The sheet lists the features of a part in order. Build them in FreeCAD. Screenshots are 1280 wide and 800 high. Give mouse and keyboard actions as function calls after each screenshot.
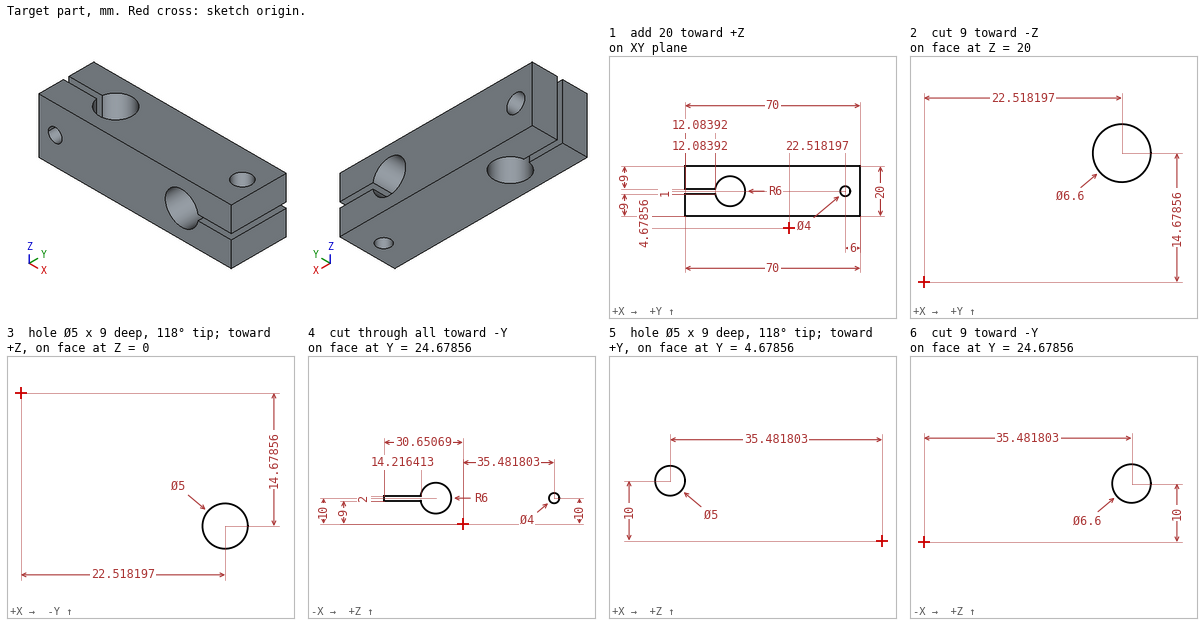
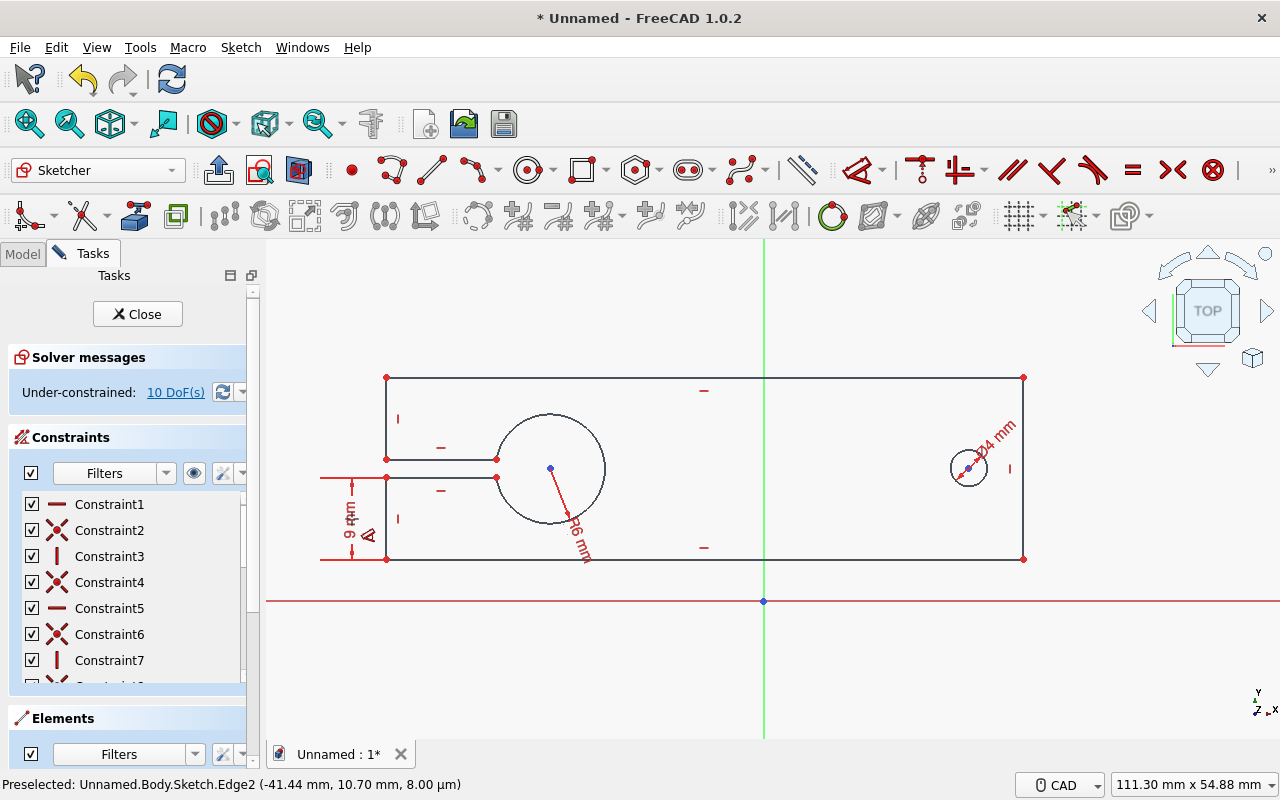
click(386, 403)
click(352, 419)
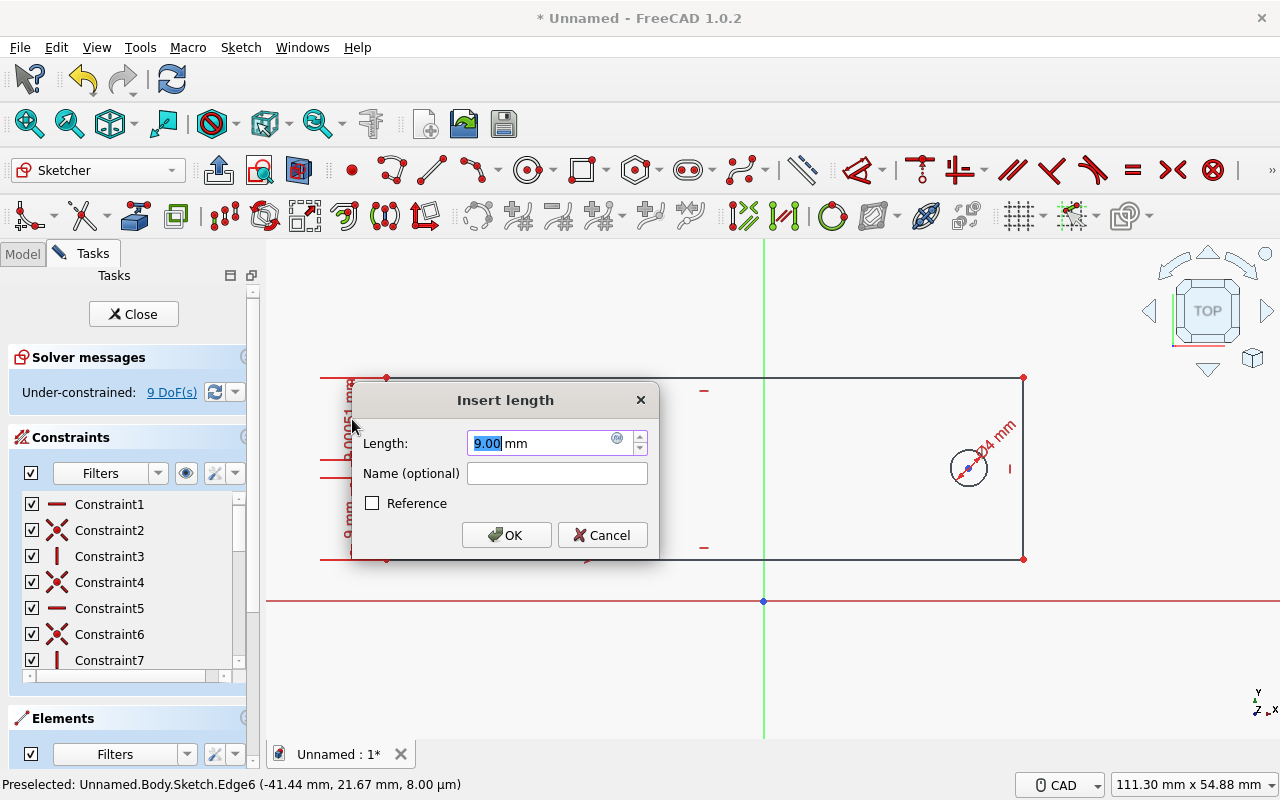
text(9)
key(Return)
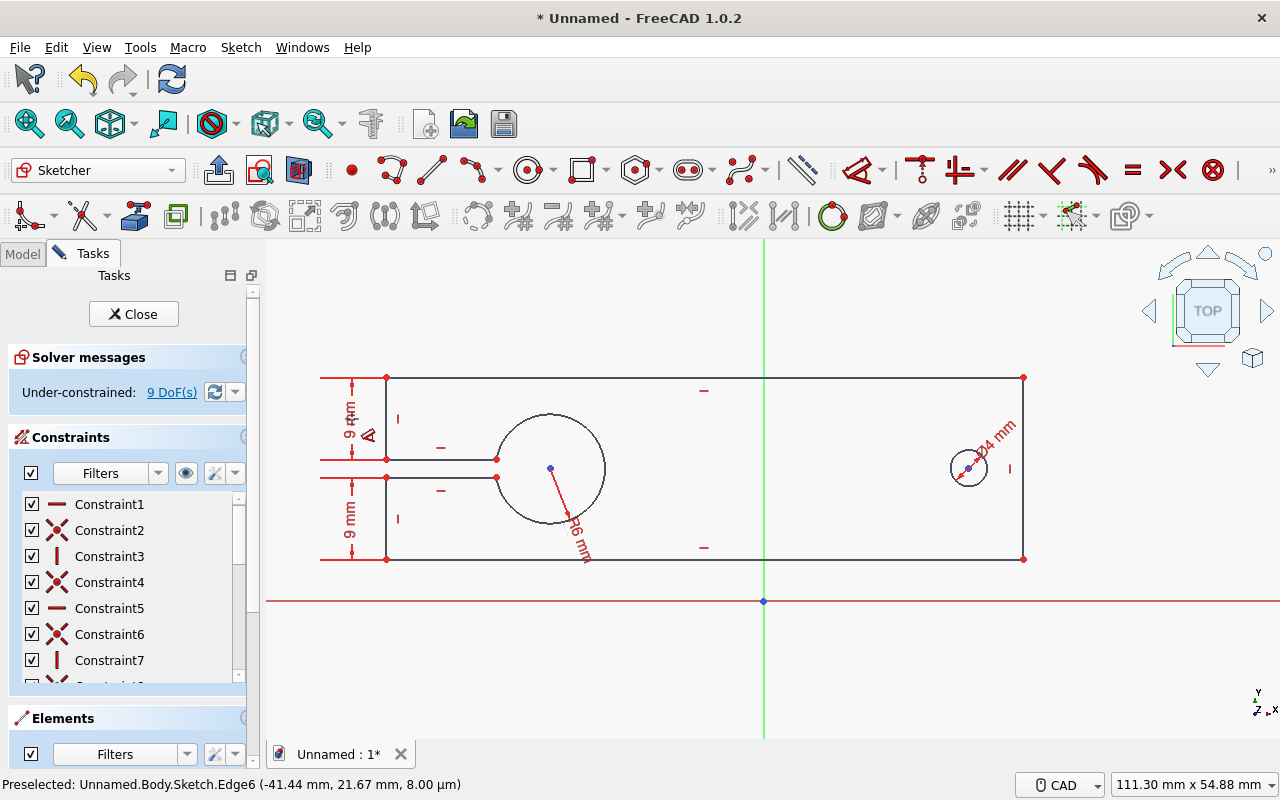
click(577, 560)
click(705, 526)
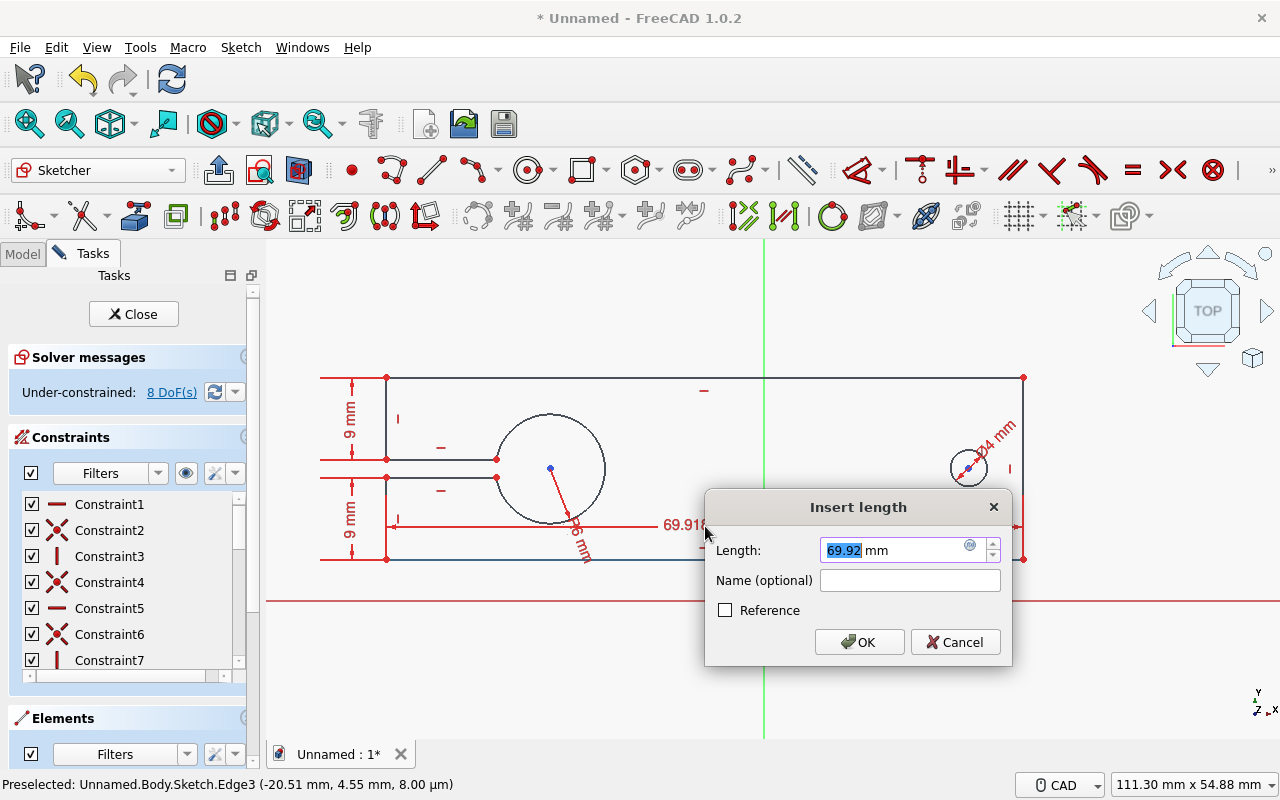
text(70)
key(Return)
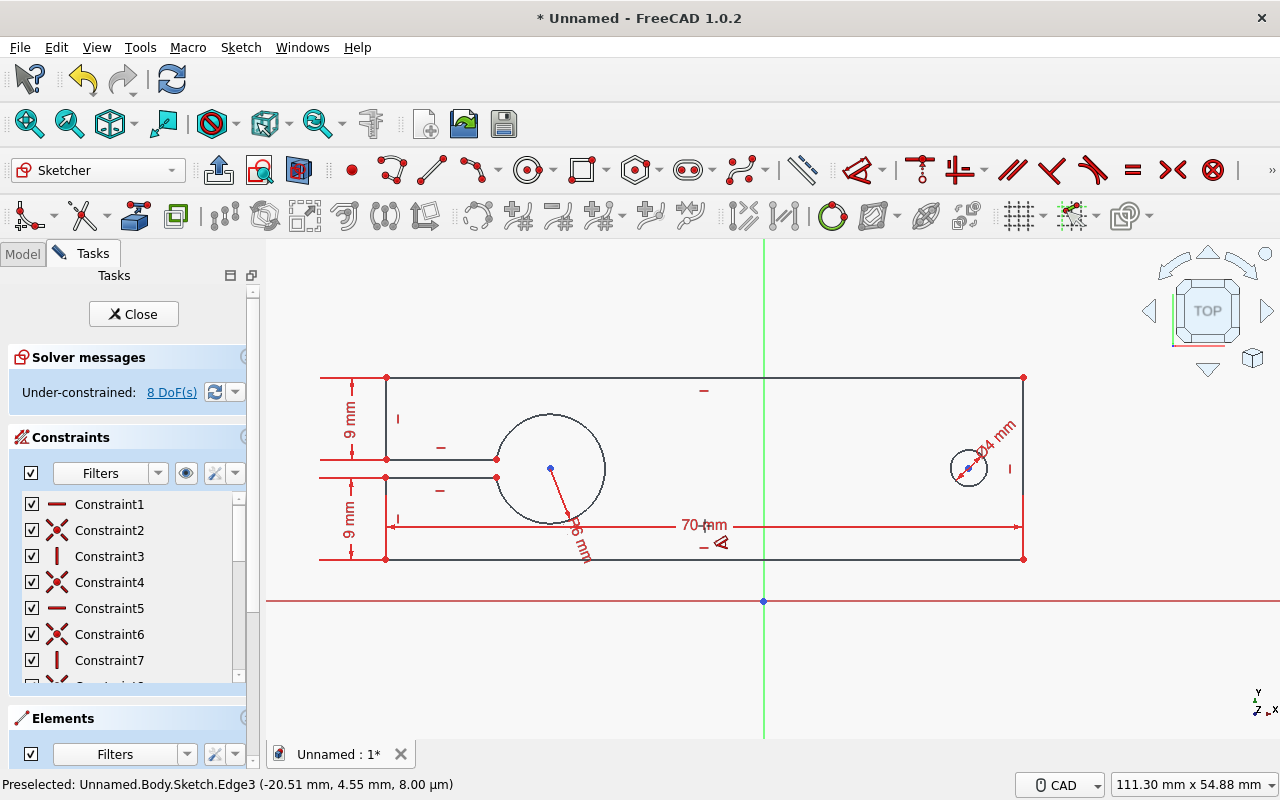
click(1023, 505)
click(1057, 469)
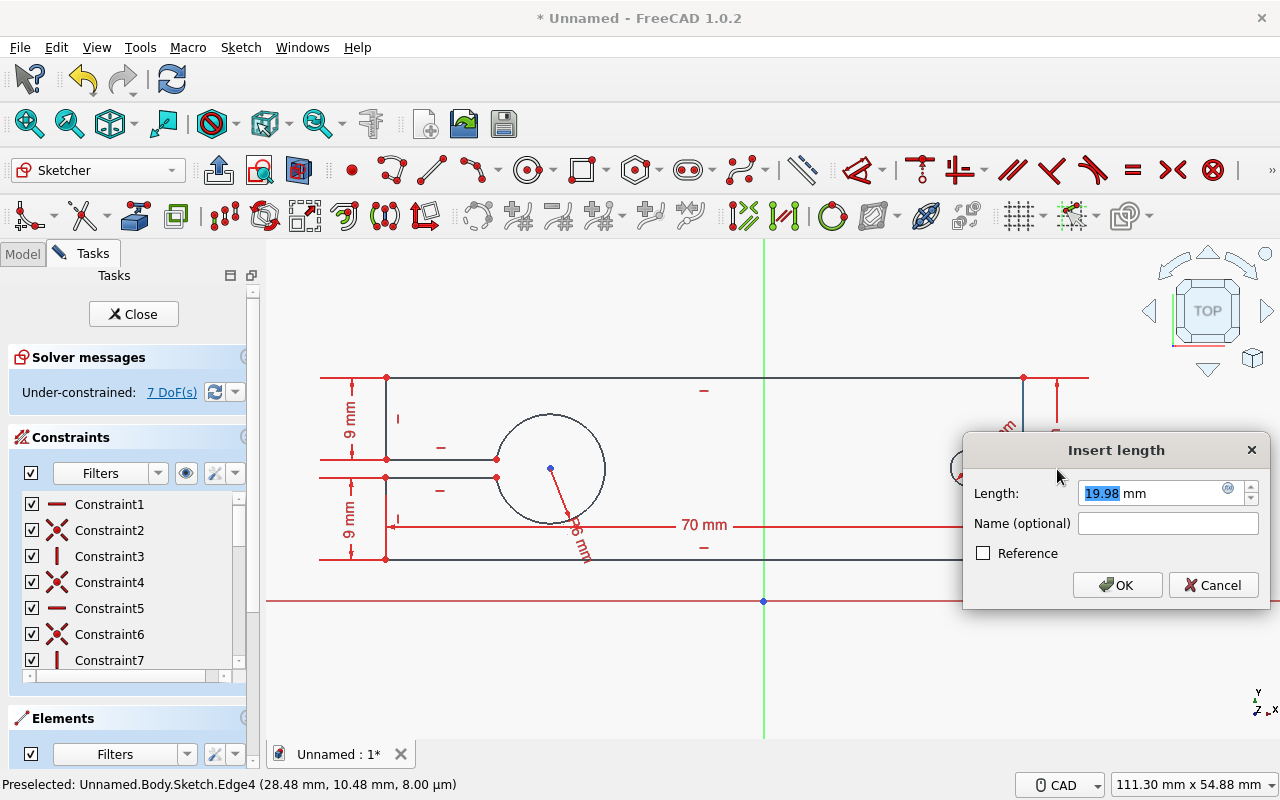
text(20)
key(Return)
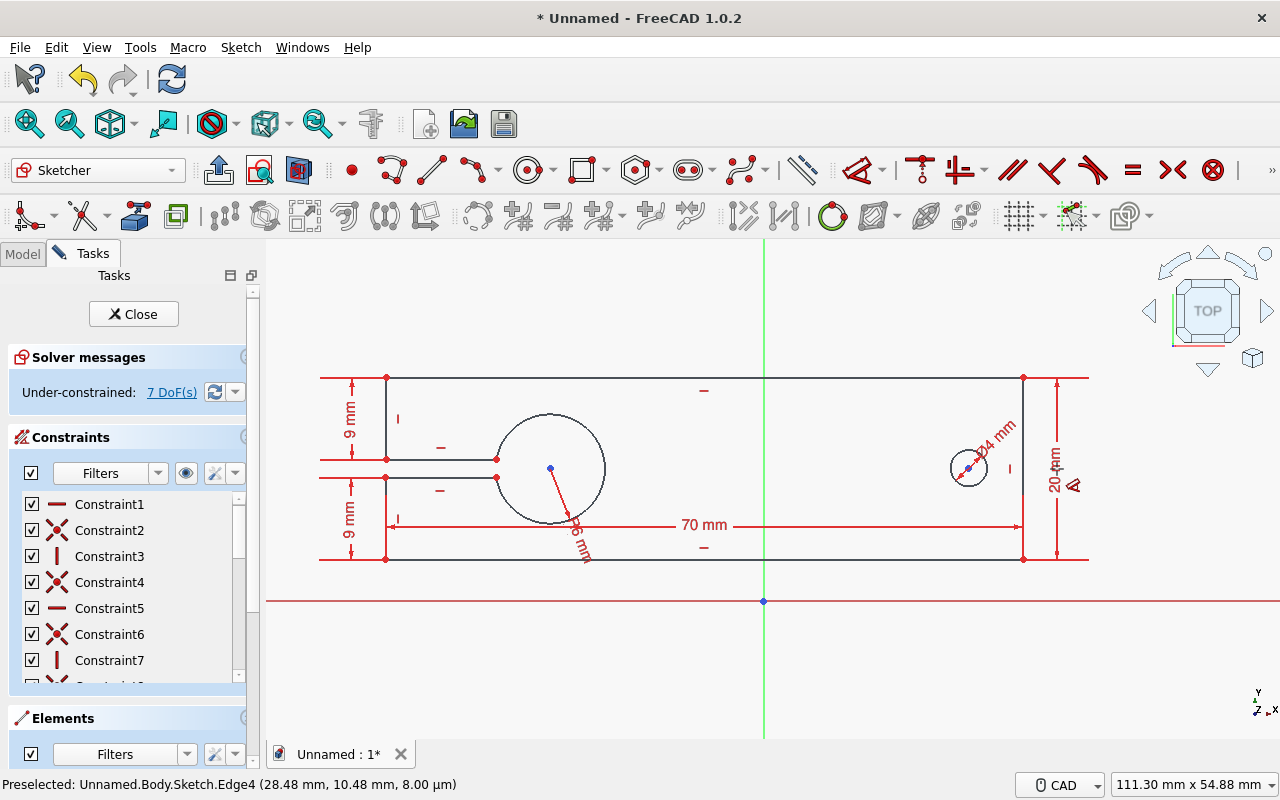
click(832, 378)
click(705, 344)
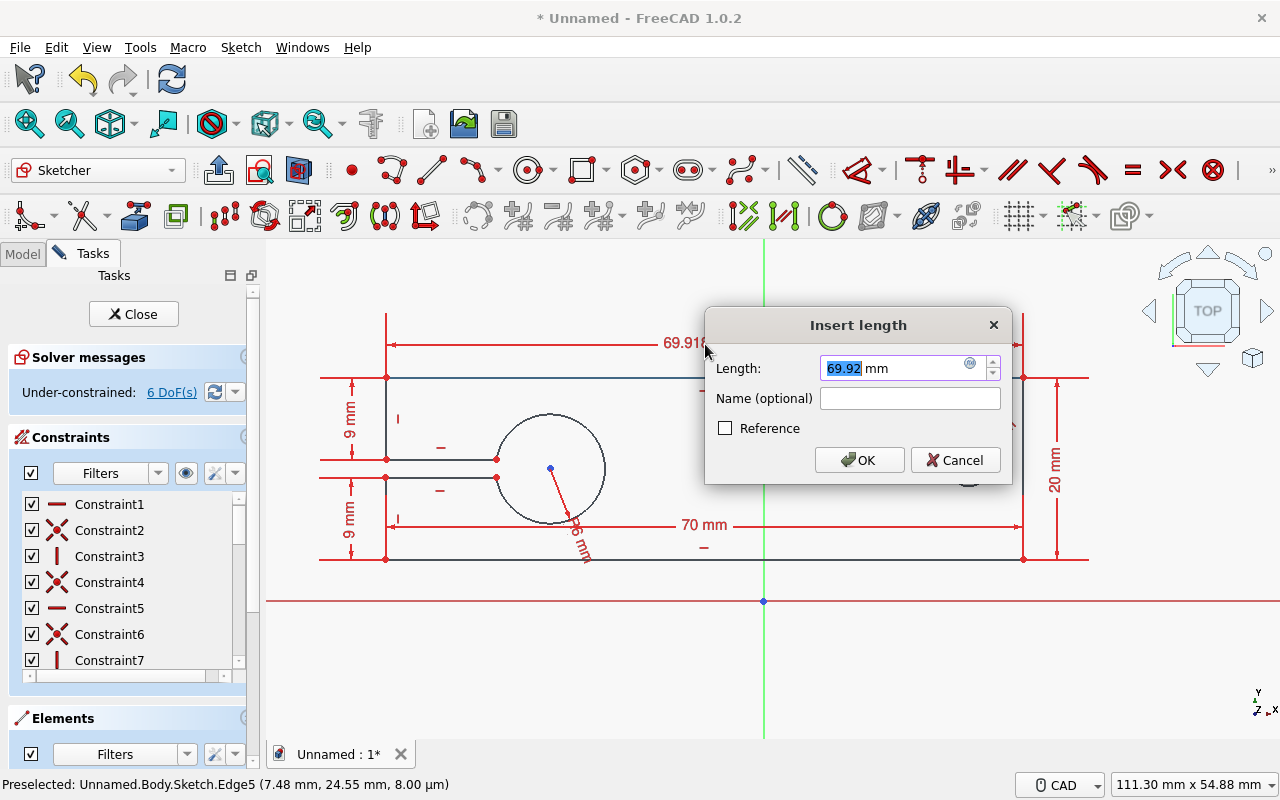
text(70)
key(Return)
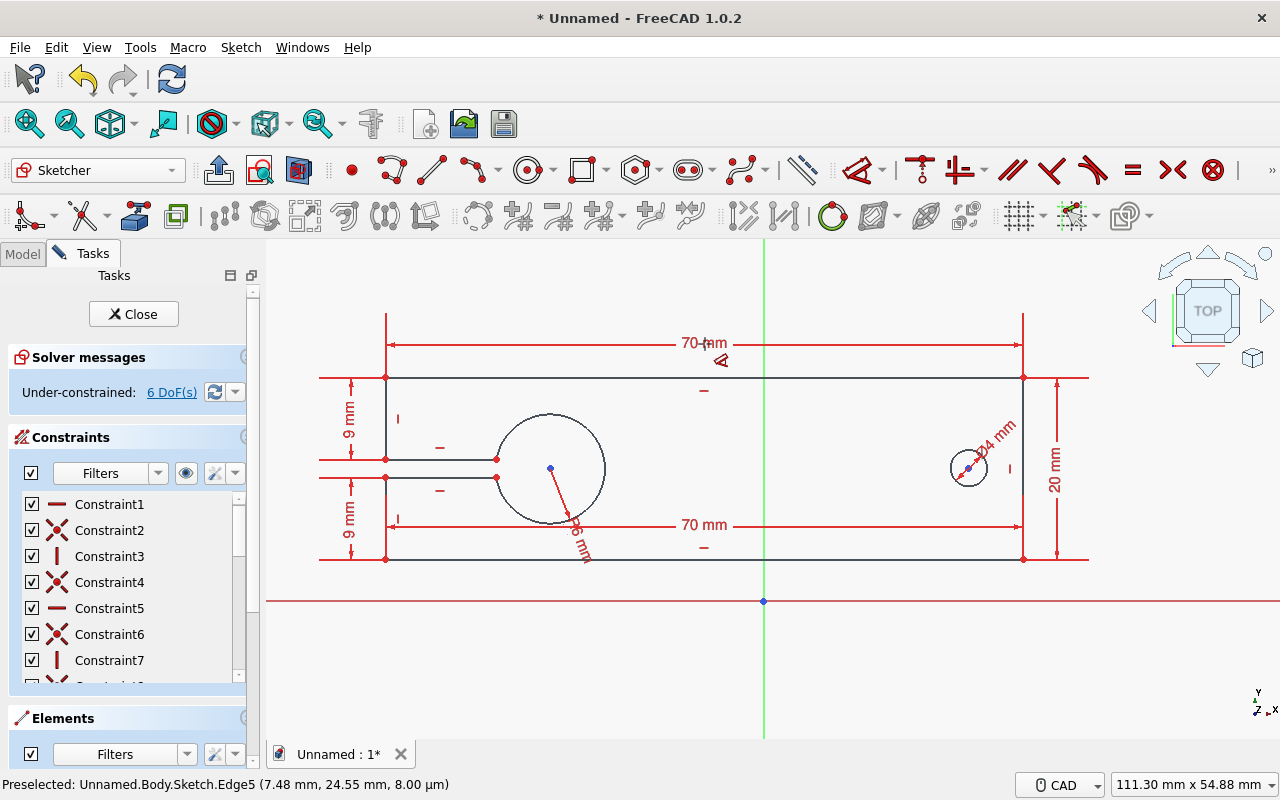
click(1023, 560)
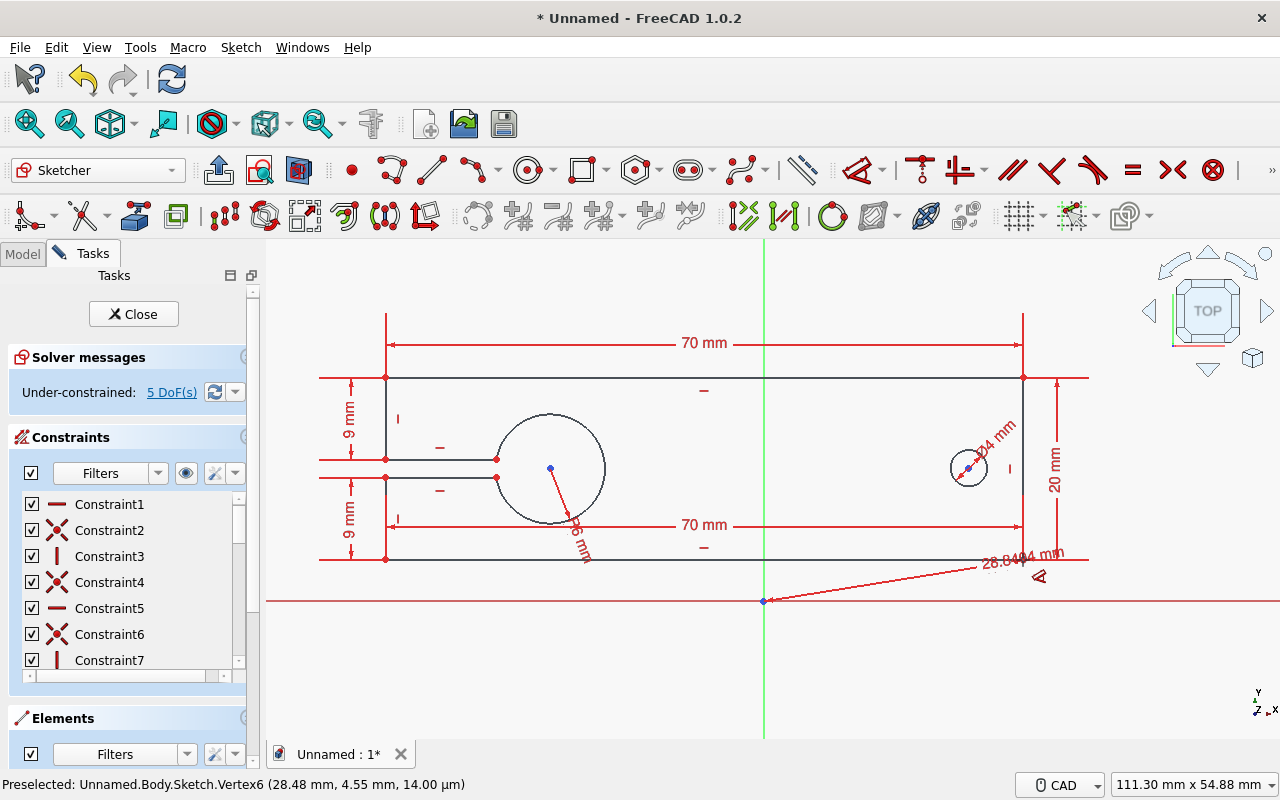
click(969, 468)
click(996, 618)